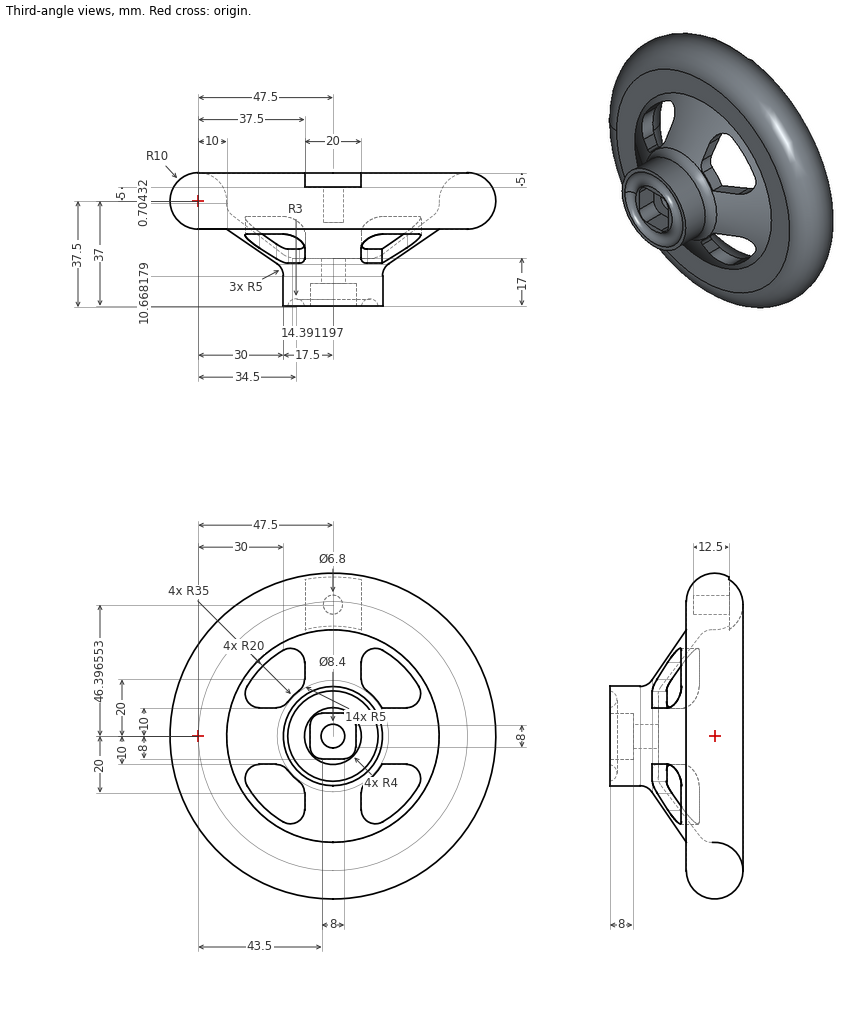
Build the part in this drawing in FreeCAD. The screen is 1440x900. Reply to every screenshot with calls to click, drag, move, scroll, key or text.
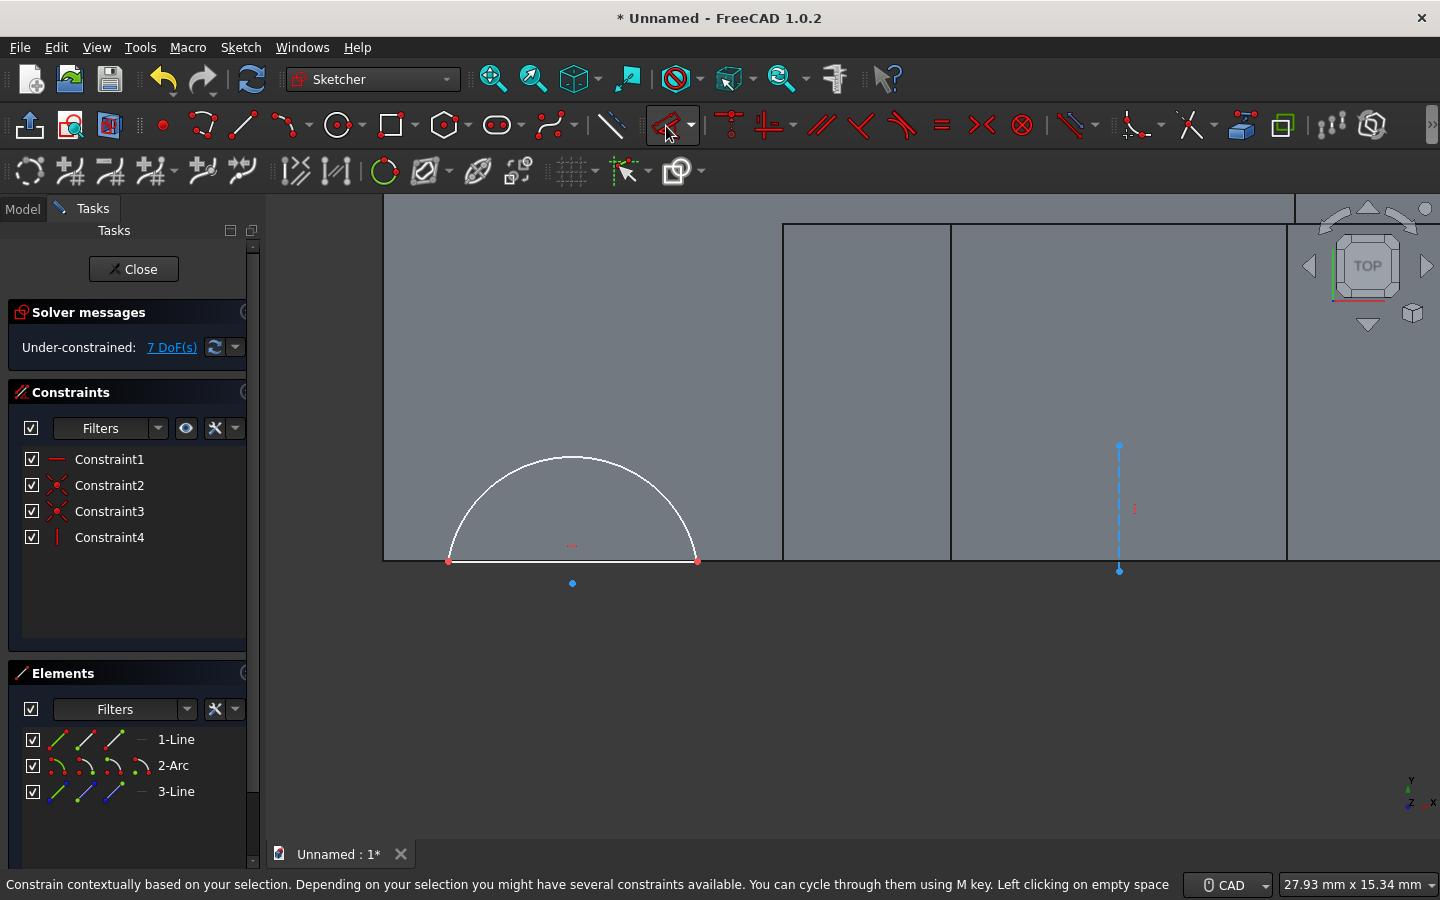
click(640, 476)
click(657, 449)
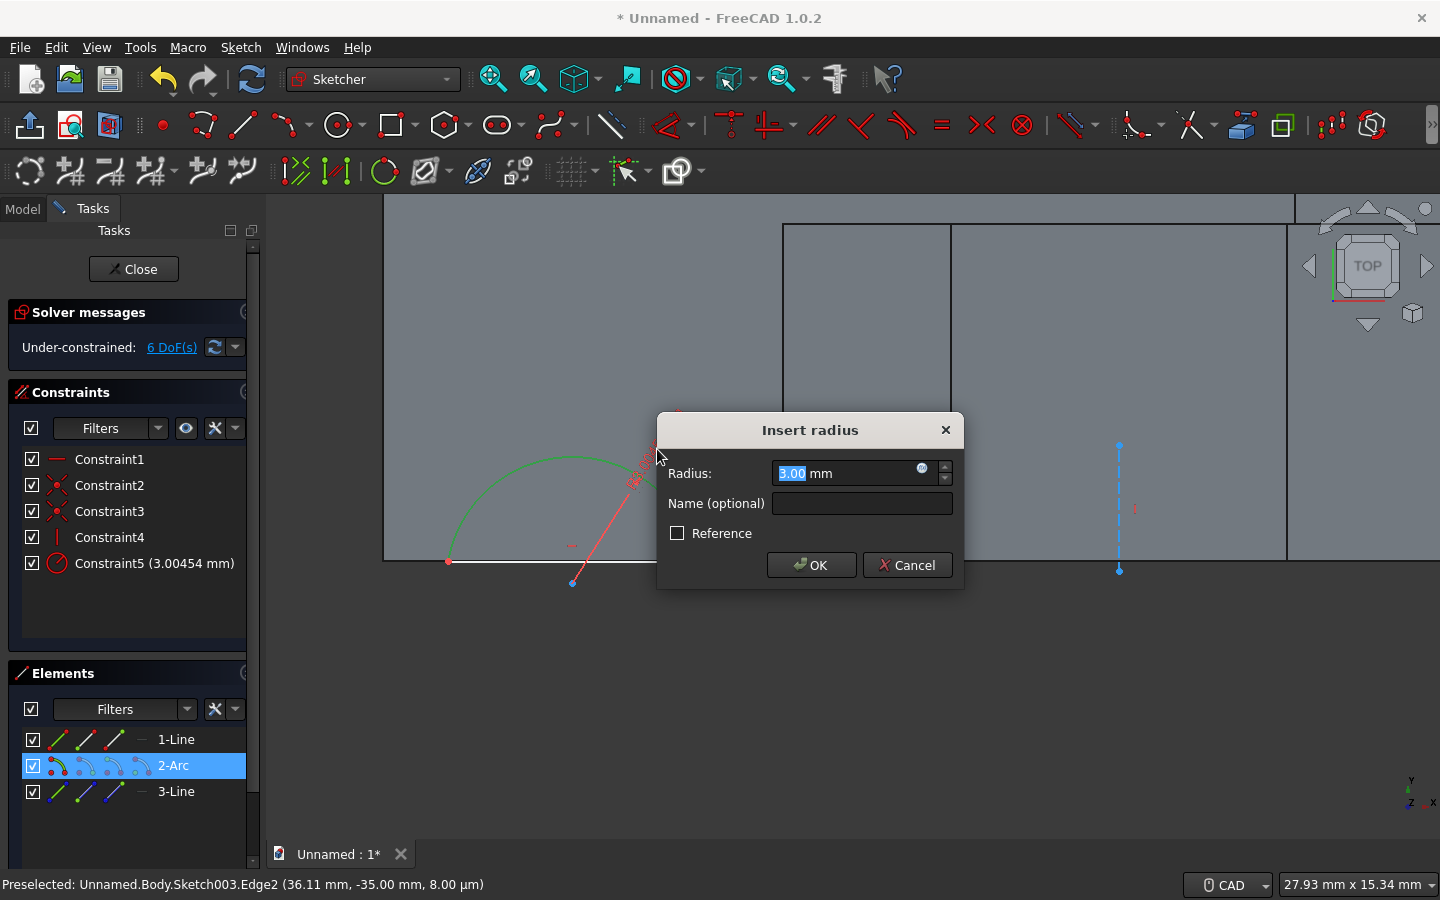
text(3)
key(Return)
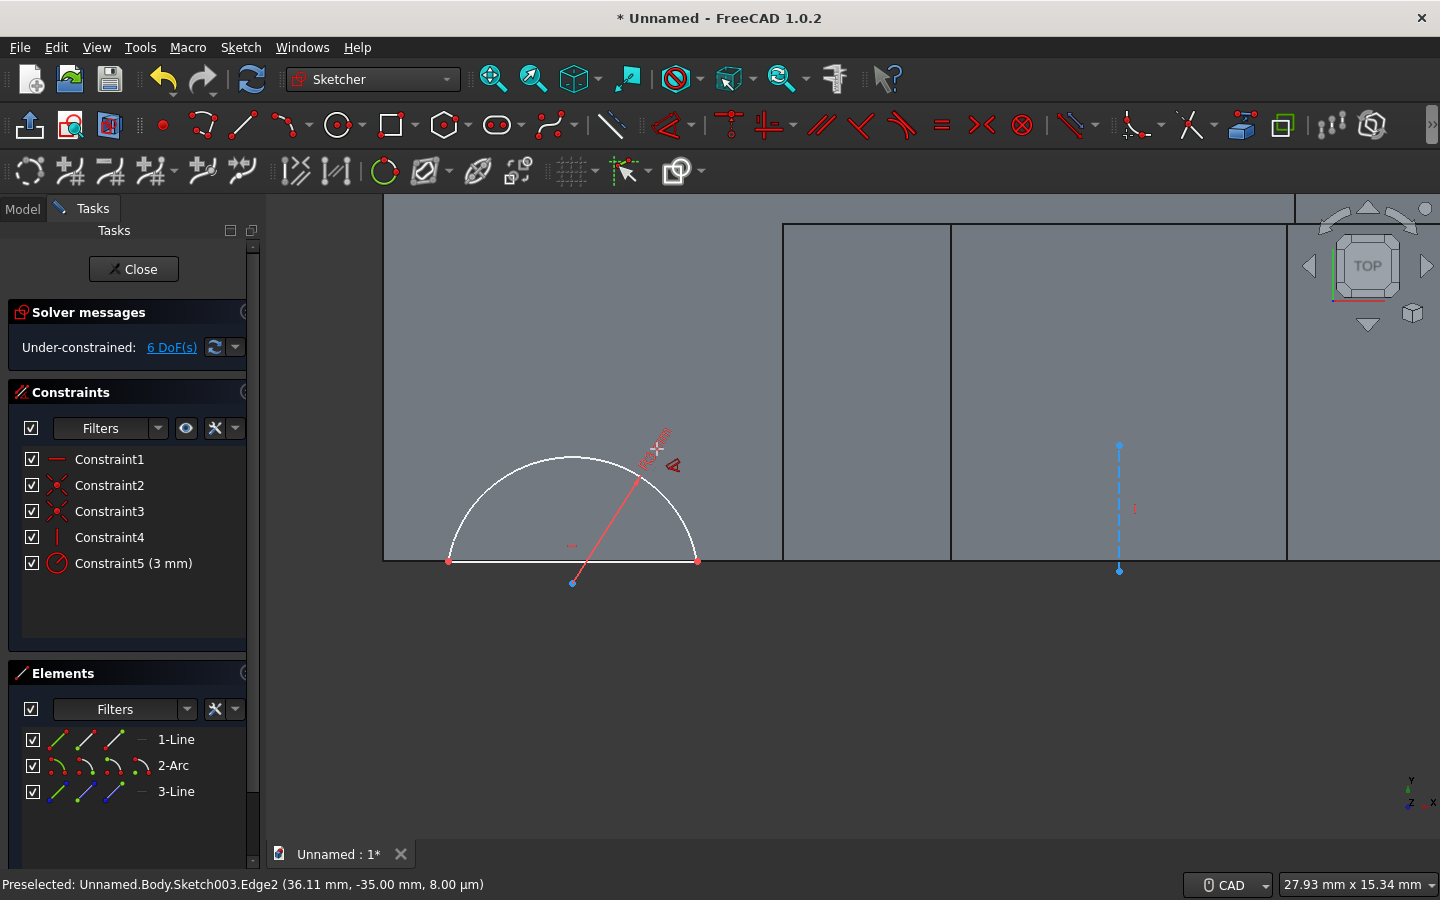
click(448, 562)
click(482, 392)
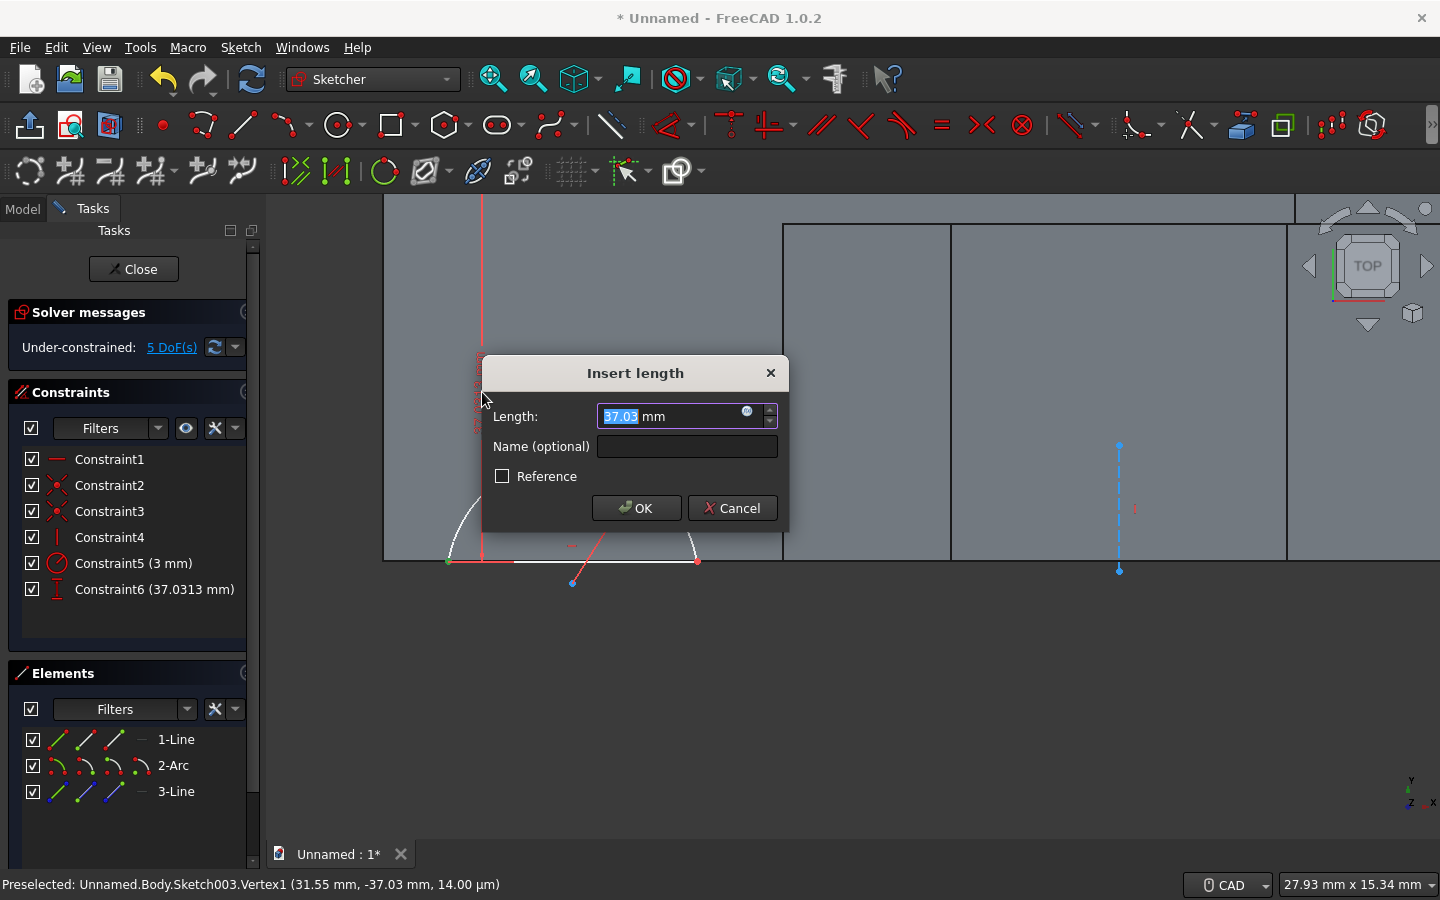
text(37)
key(Return)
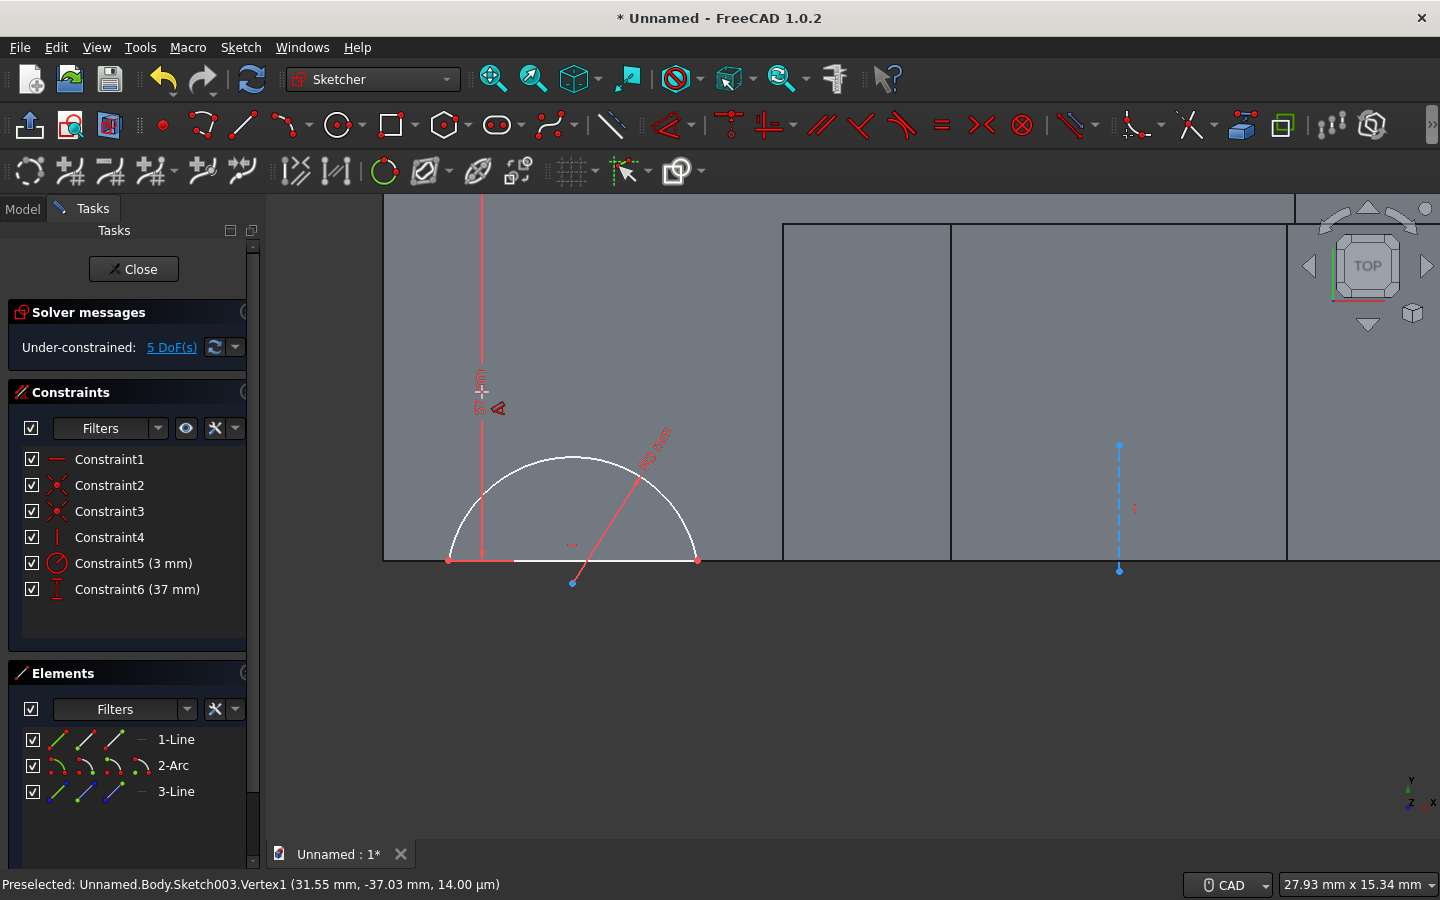
click(1119, 446)
click(707, 480)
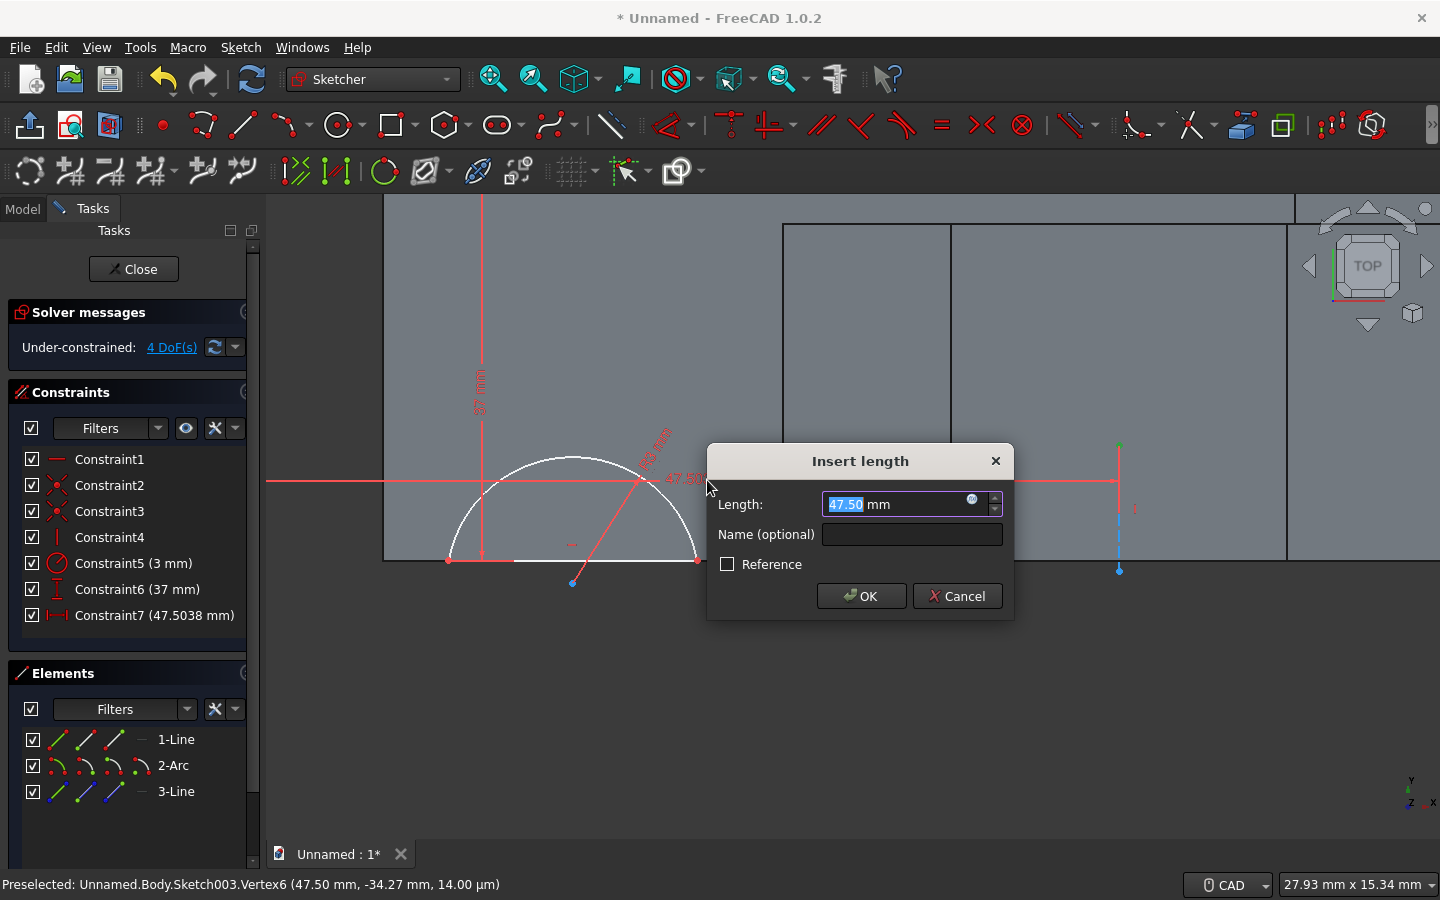
text(47.5)
key(Return)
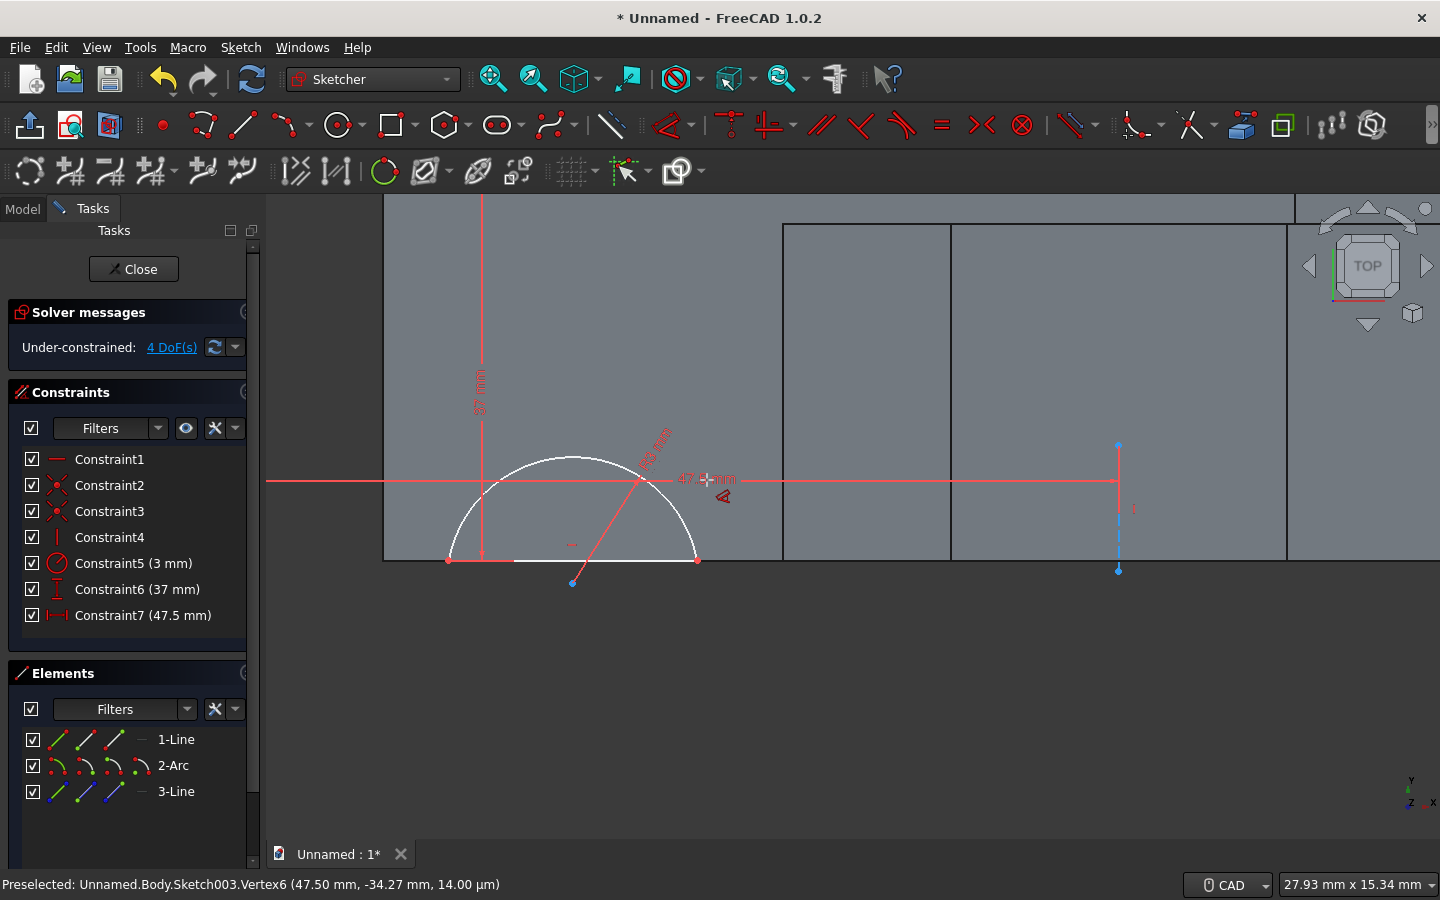
click(573, 583)
click(433, 617)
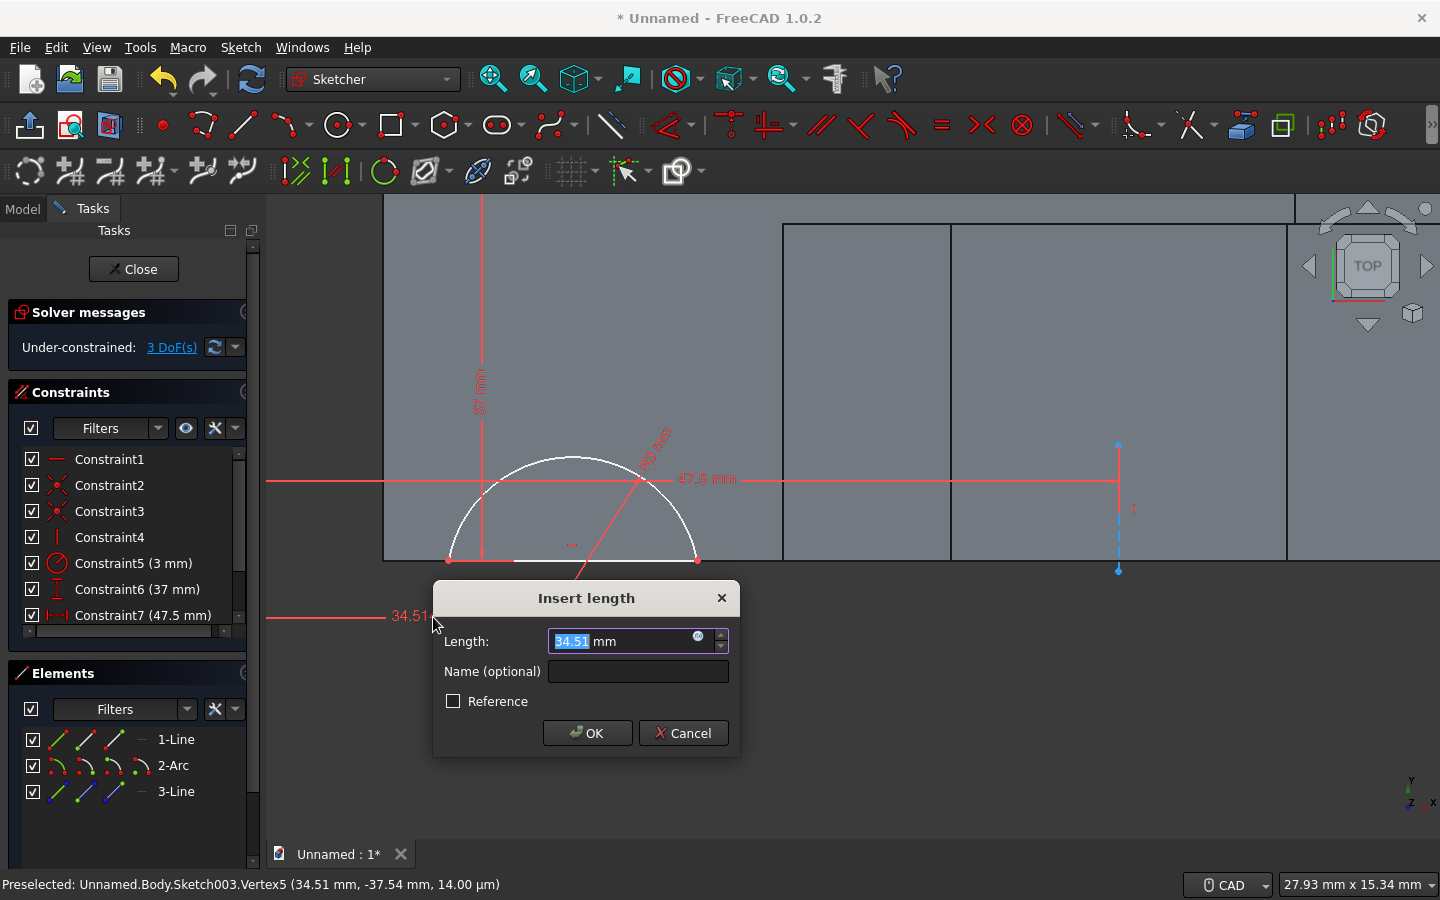
text(34.5)
key(Return)